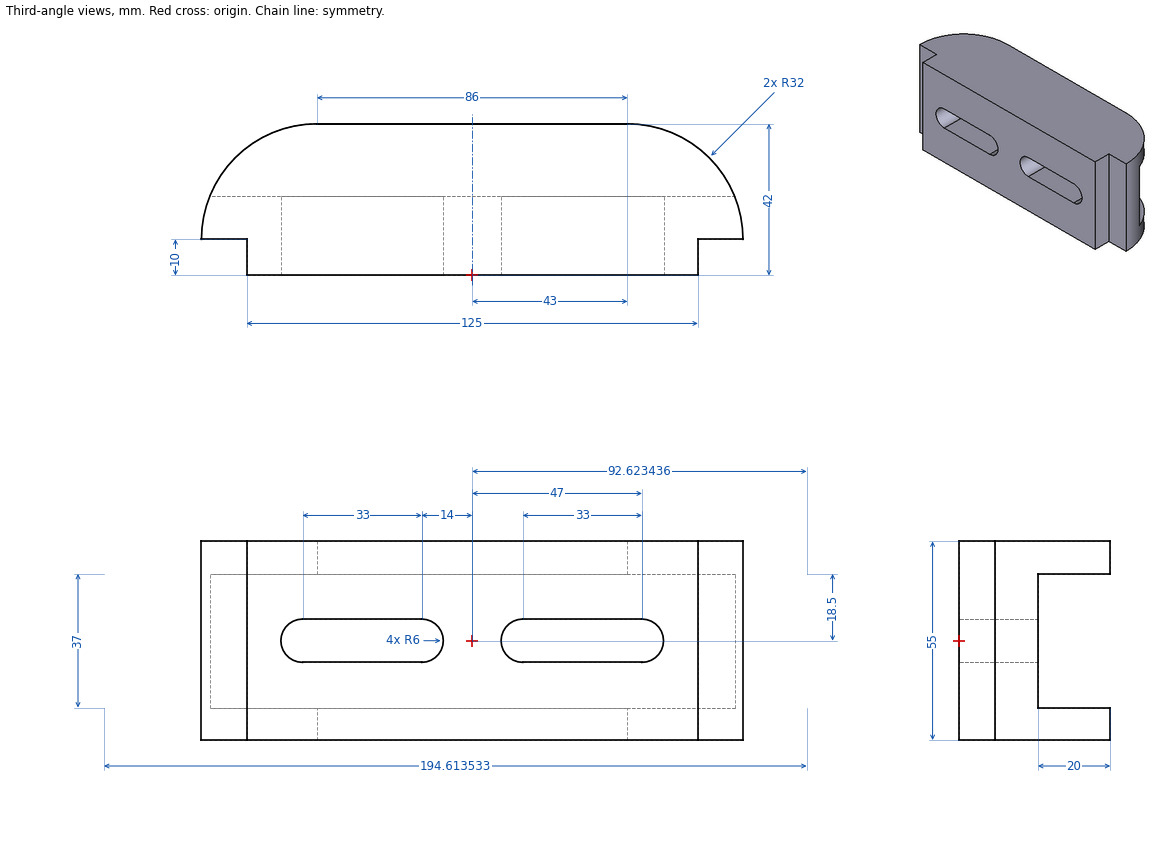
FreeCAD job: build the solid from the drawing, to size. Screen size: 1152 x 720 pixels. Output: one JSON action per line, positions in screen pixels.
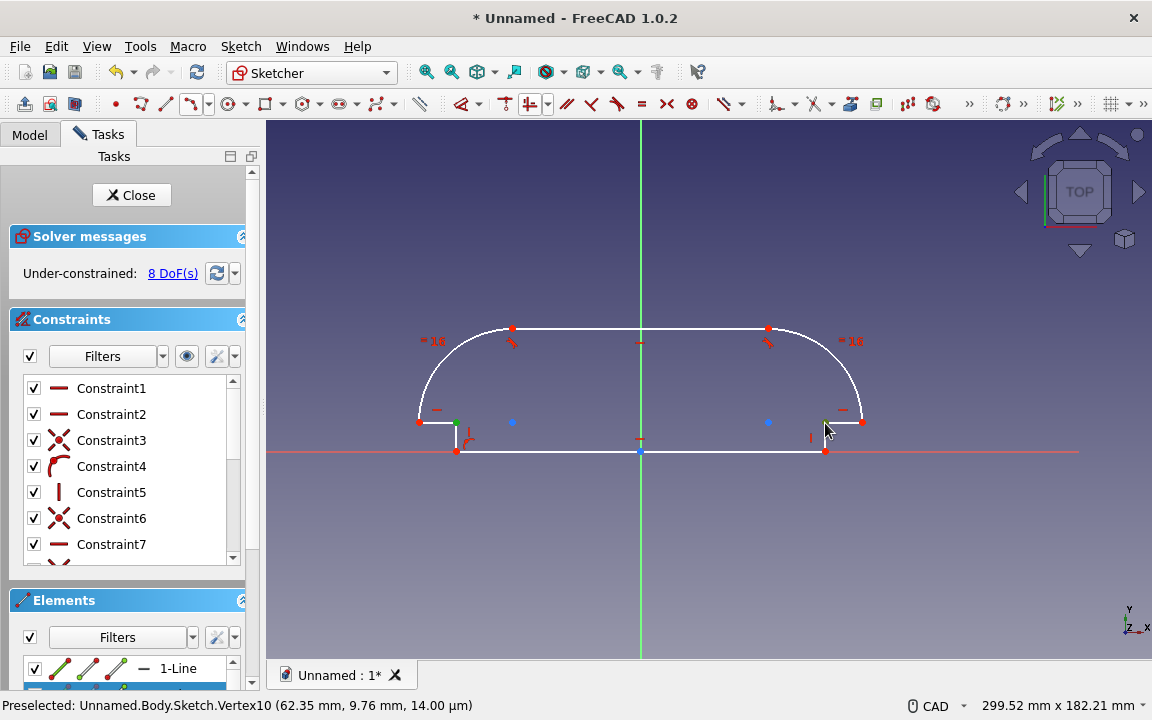
{"action": "left_click", "coordinate": [641, 596]}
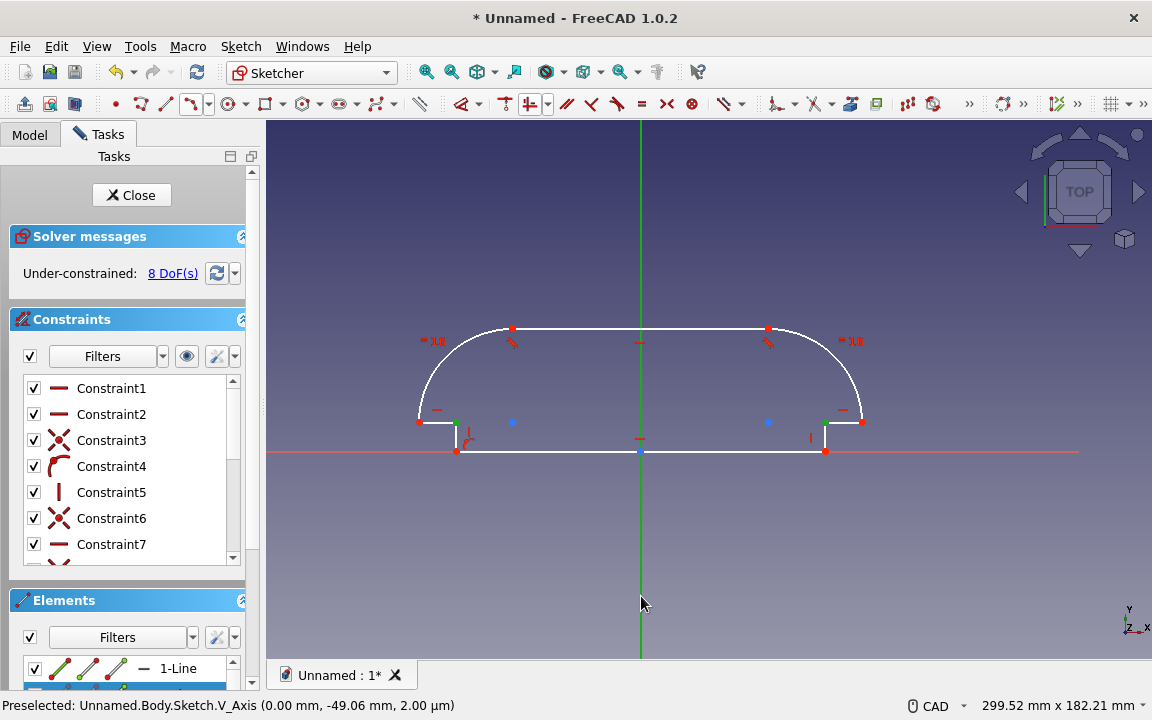
{"action": "left_click", "coordinate": [667, 104]}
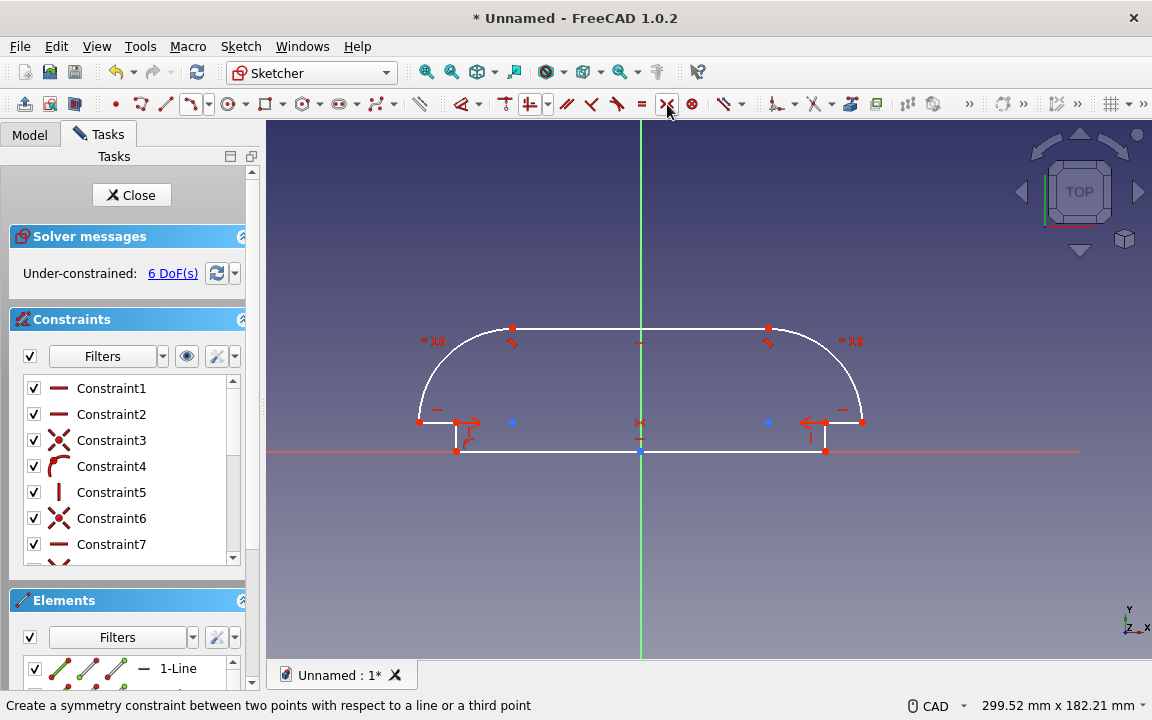
{"action": "left_click", "coordinate": [460, 104]}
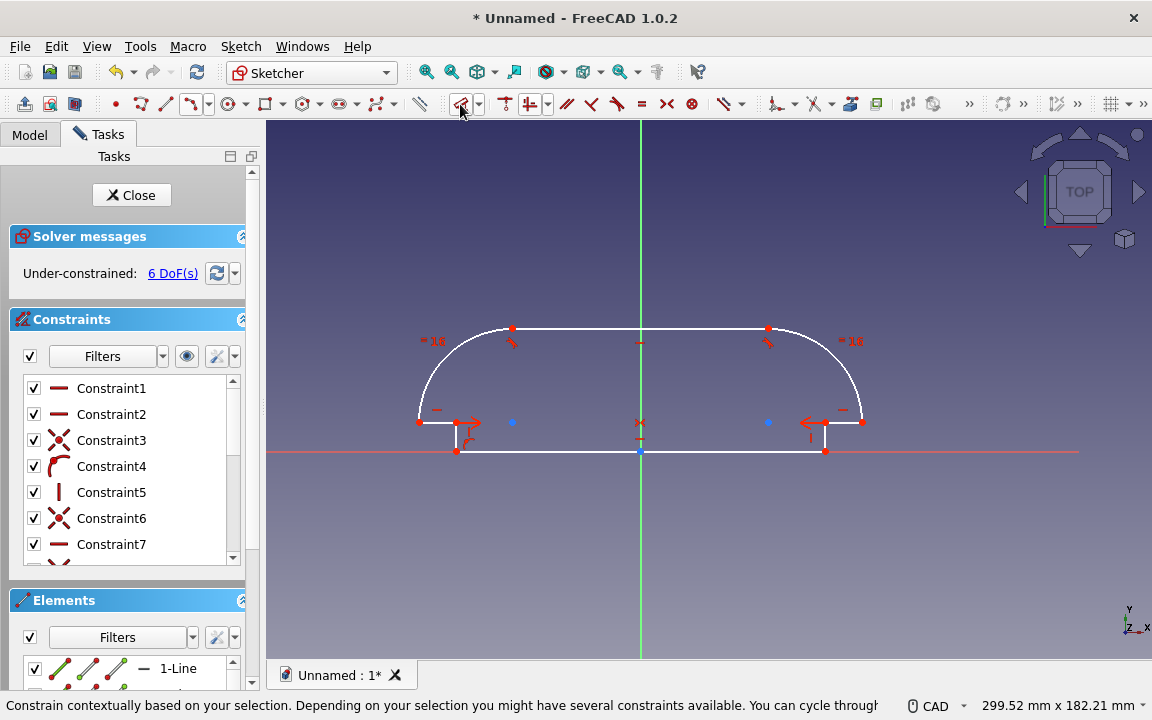
{"action": "left_click", "coordinate": [470, 339]}
{"action": "left_click", "coordinate": [455, 311]}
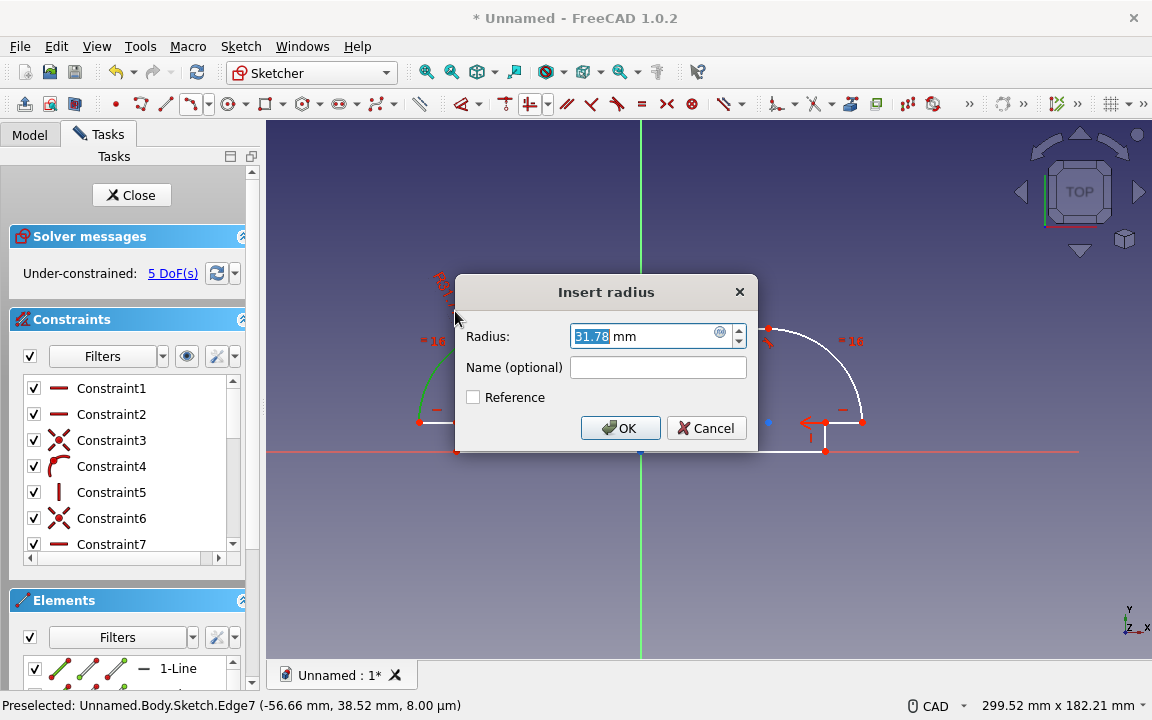
{"action": "type", "text": "32"}
{"action": "key", "text": "Return"}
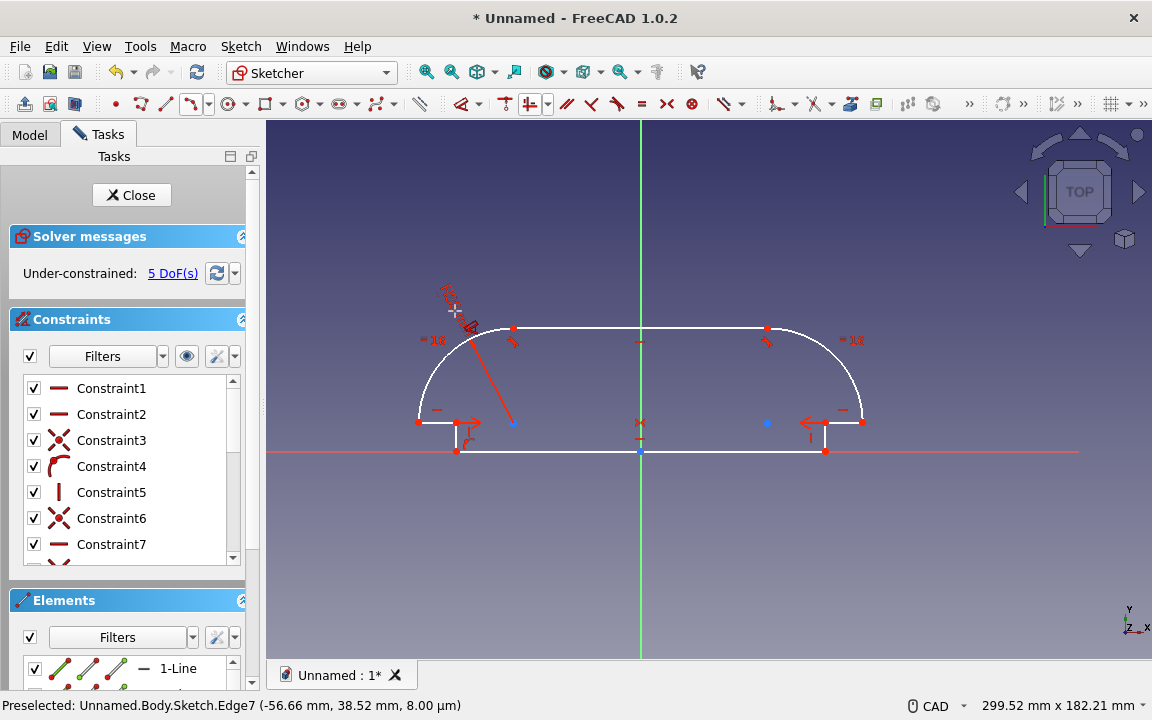
{"action": "left_click", "coordinate": [692, 328]}
{"action": "left_click", "coordinate": [582, 294]}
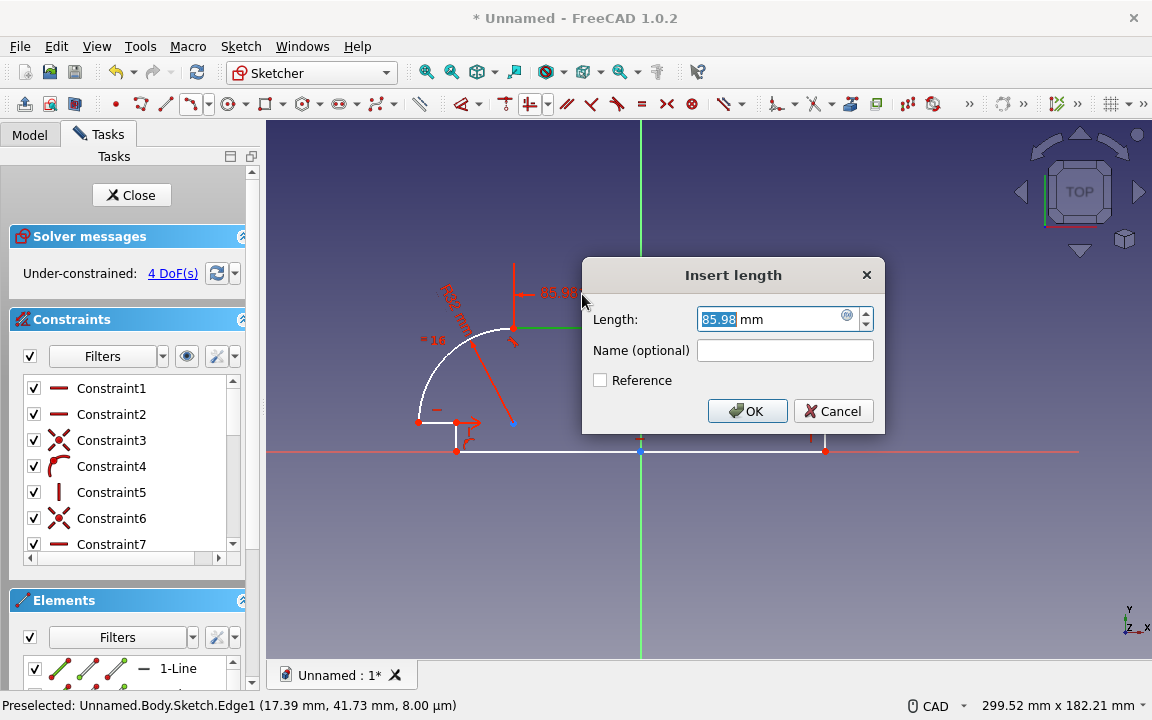
{"action": "type", "text": "86"}
{"action": "key", "text": "Return"}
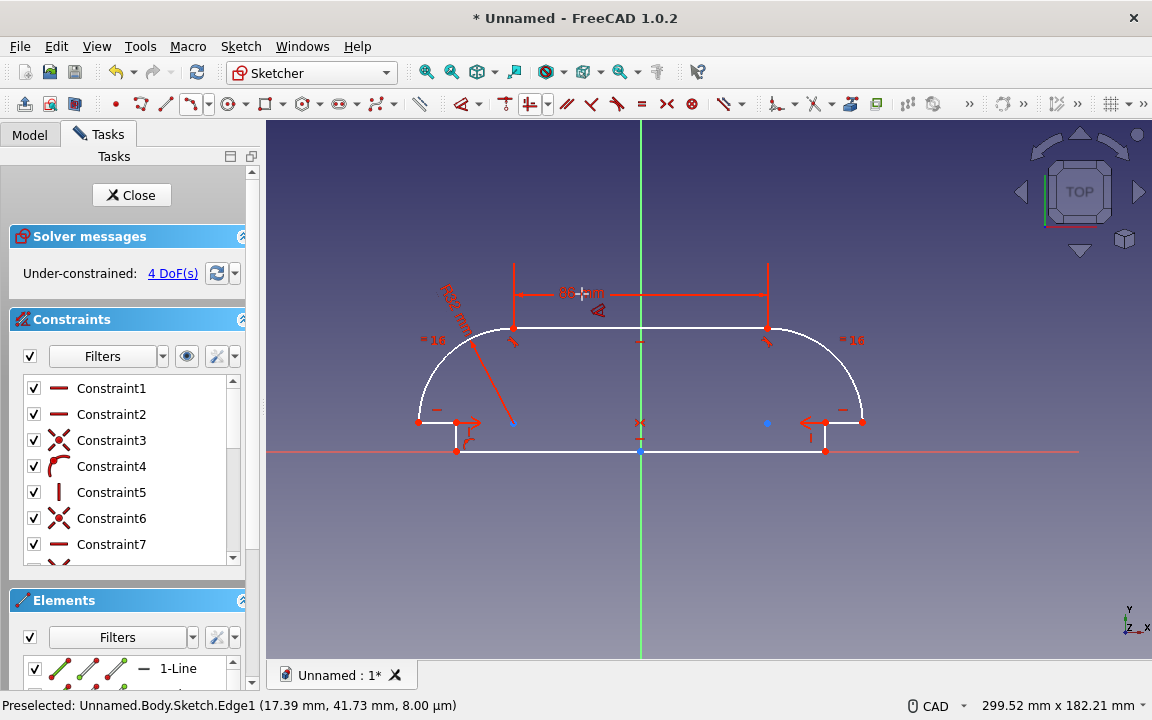
{"action": "scroll", "coordinate": [456, 435], "scroll_direction": "up", "scroll_amount": 2}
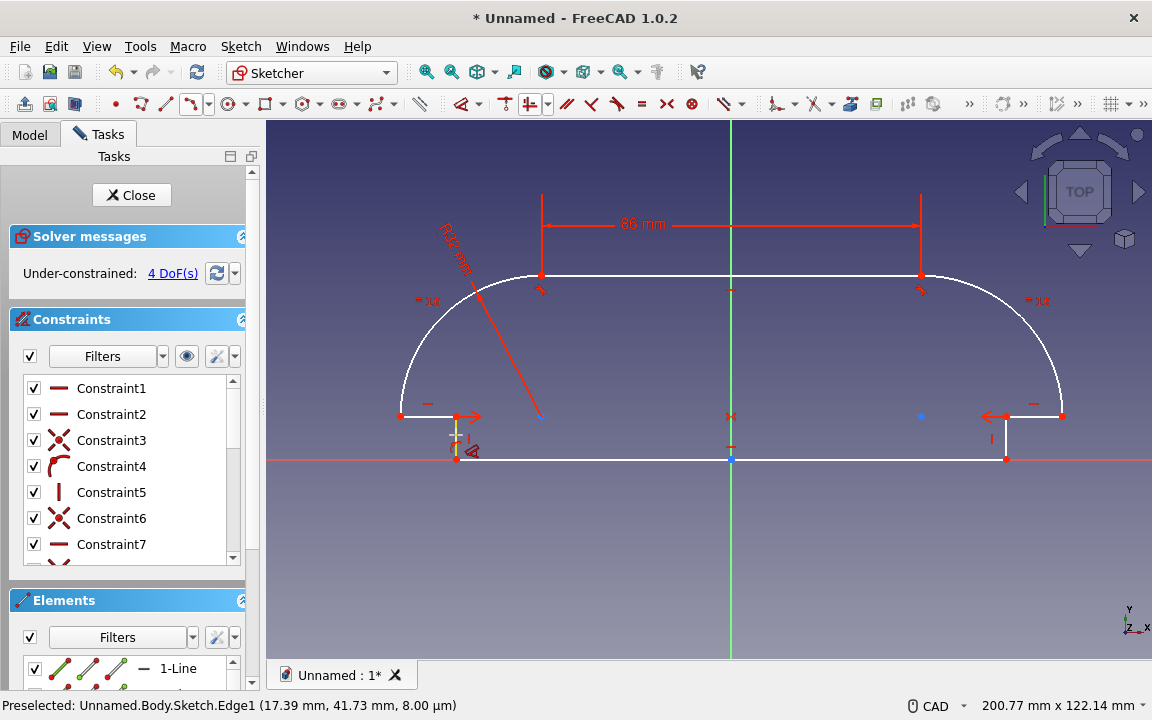
{"action": "left_click", "coordinate": [456, 434]}
{"action": "left_click", "coordinate": [422, 438]}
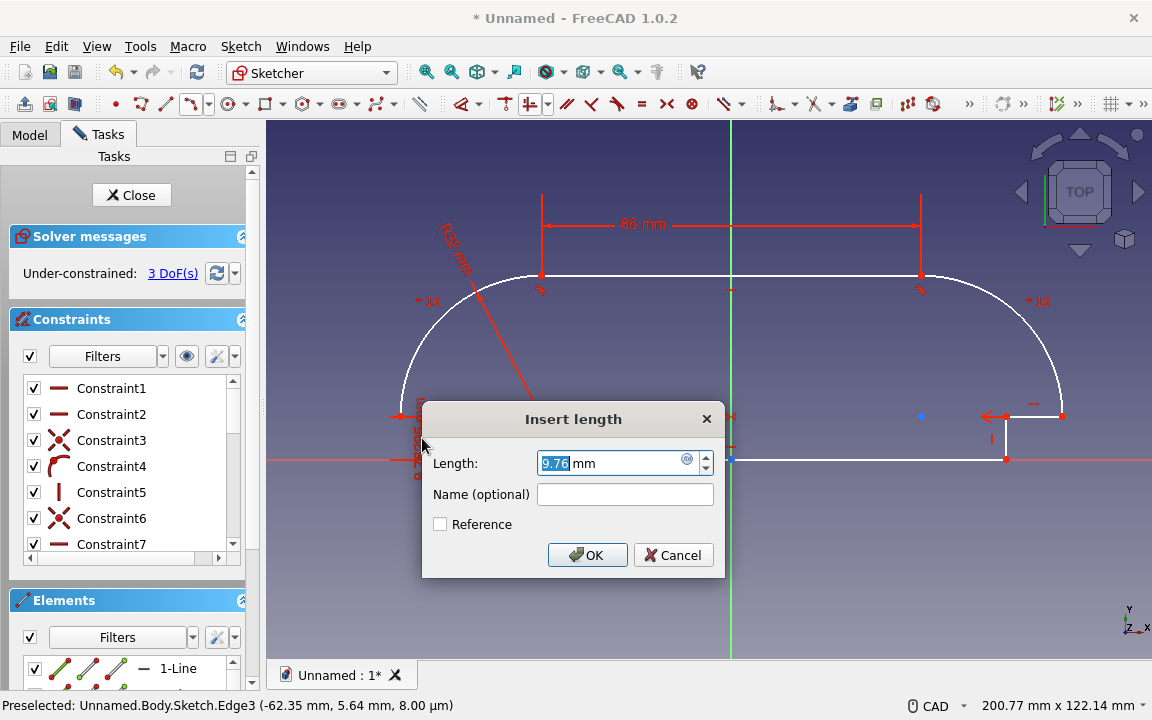
{"action": "type", "text": "10"}
{"action": "key", "text": "Return"}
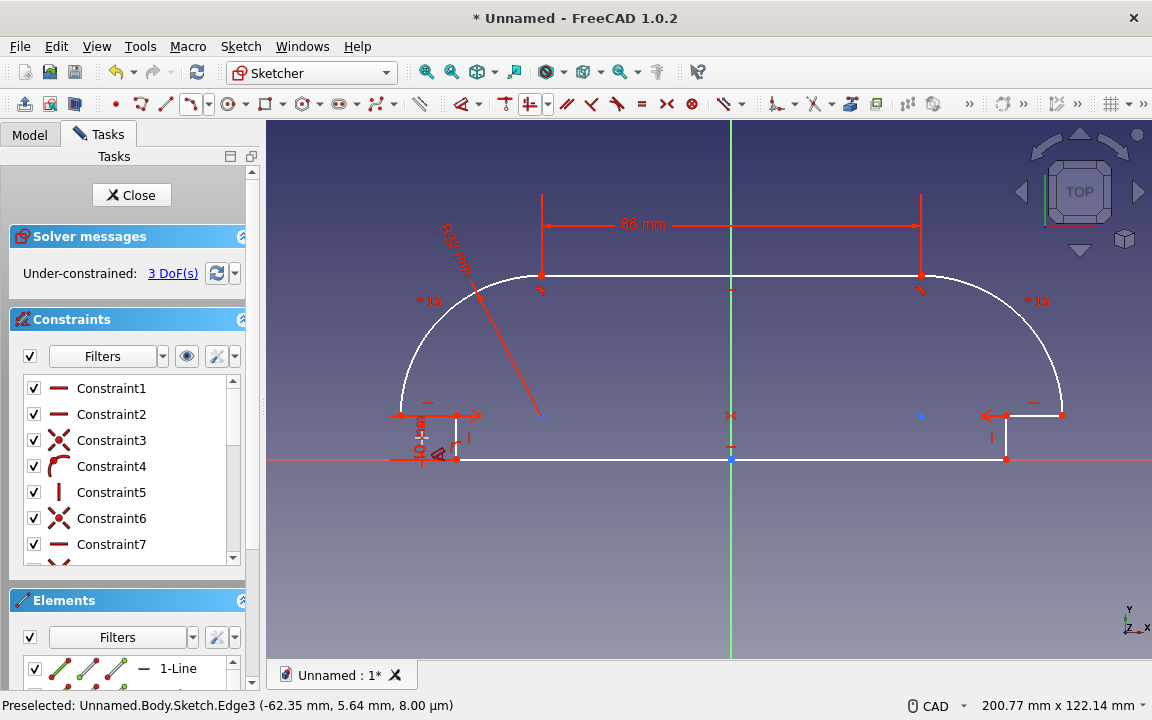
{"action": "left_click", "coordinate": [621, 460]}
{"action": "left_click", "coordinate": [599, 494]}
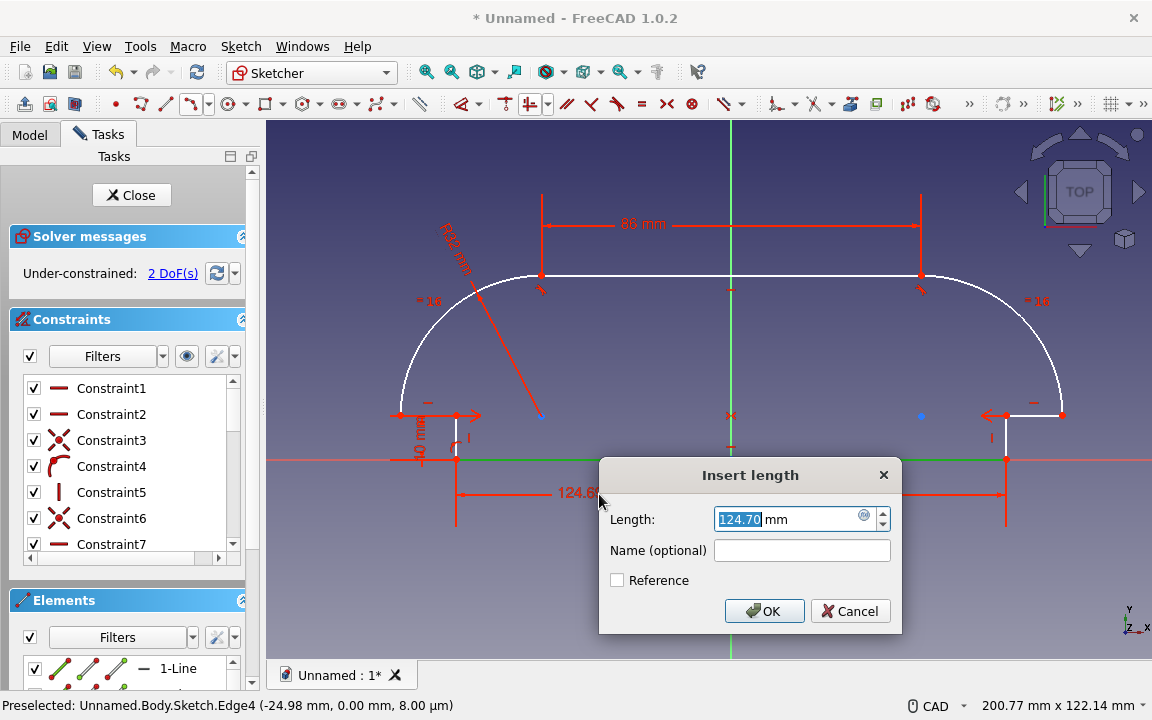
{"action": "type", "text": "125"}
{"action": "key", "text": "Return"}